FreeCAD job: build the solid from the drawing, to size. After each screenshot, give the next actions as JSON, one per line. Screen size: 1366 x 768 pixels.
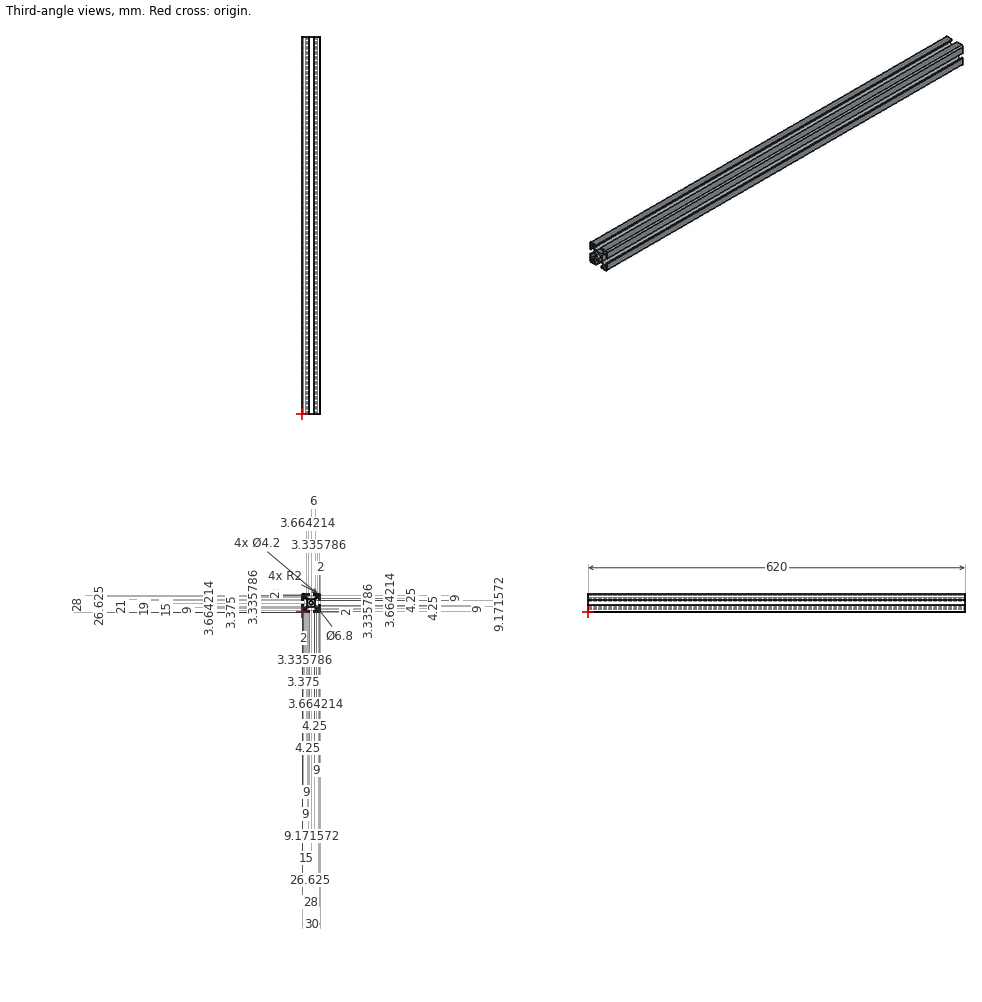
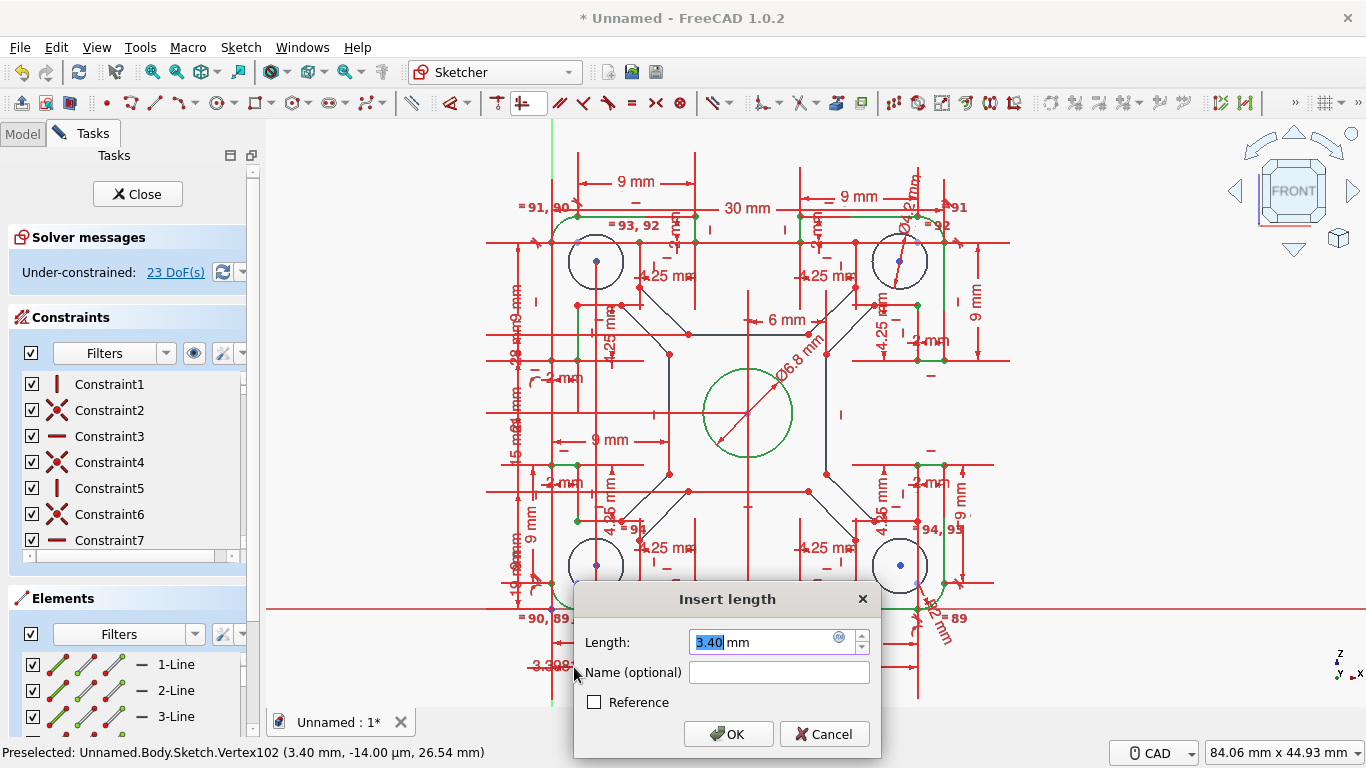
{"action": "type", "text": "3.375"}
{"action": "key", "text": "Return"}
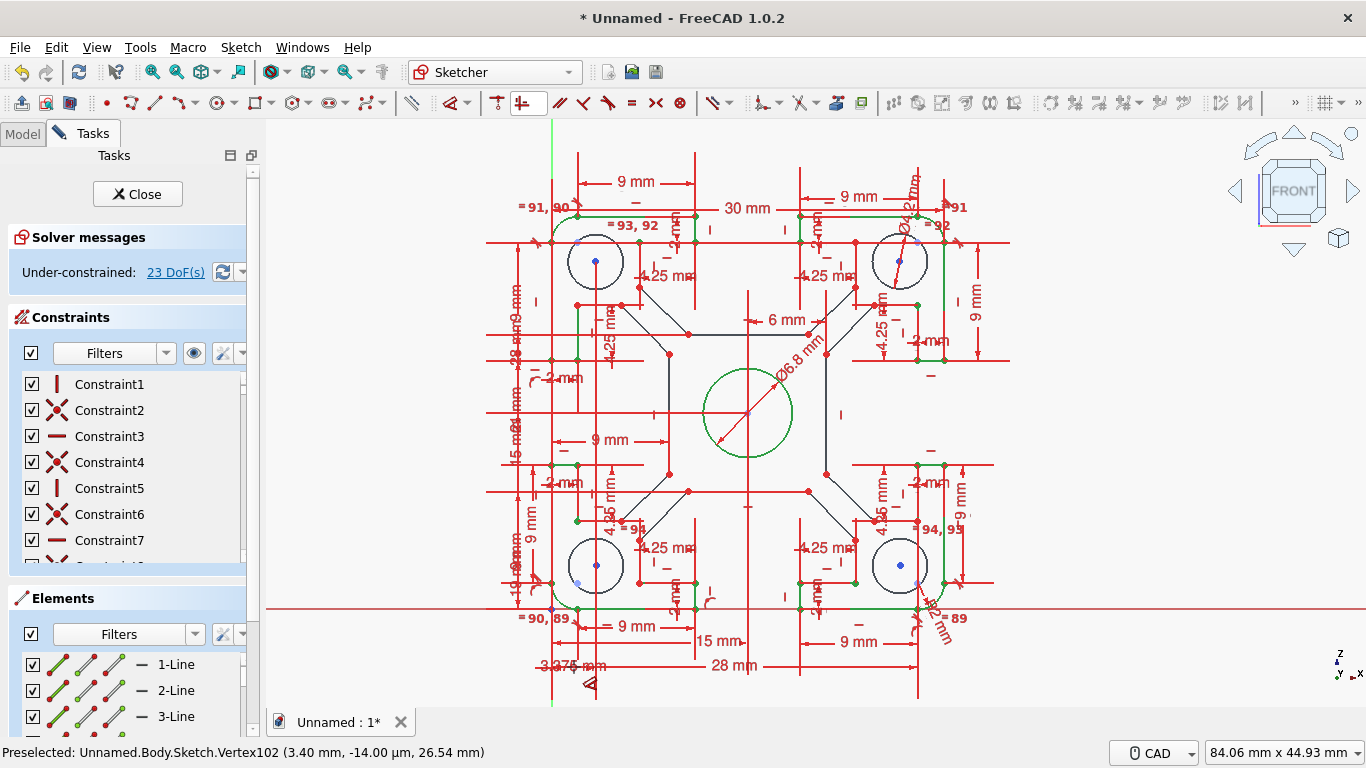
{"action": "left_click", "coordinate": [900, 566]}
{"action": "left_click", "coordinate": [958, 588]}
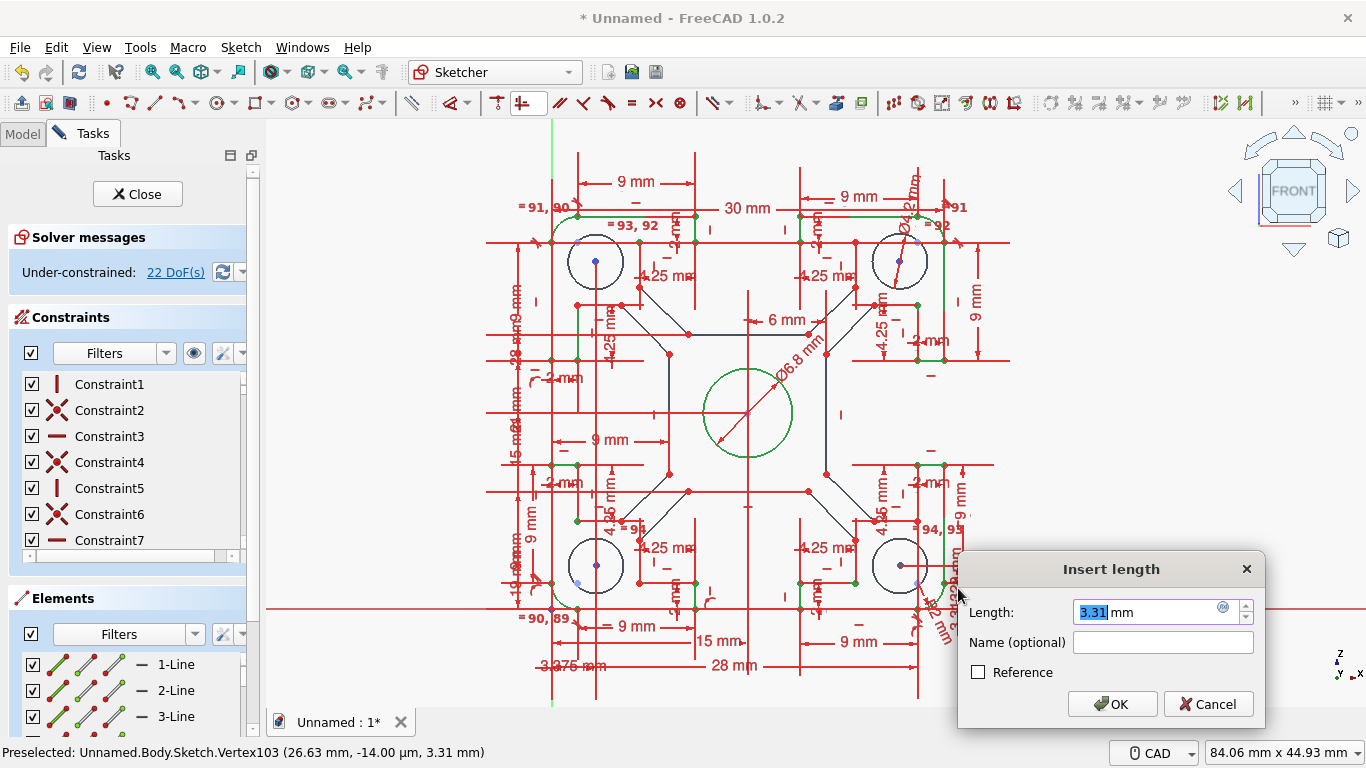
{"action": "type", "text": "3.375"}
{"action": "key", "text": "Return"}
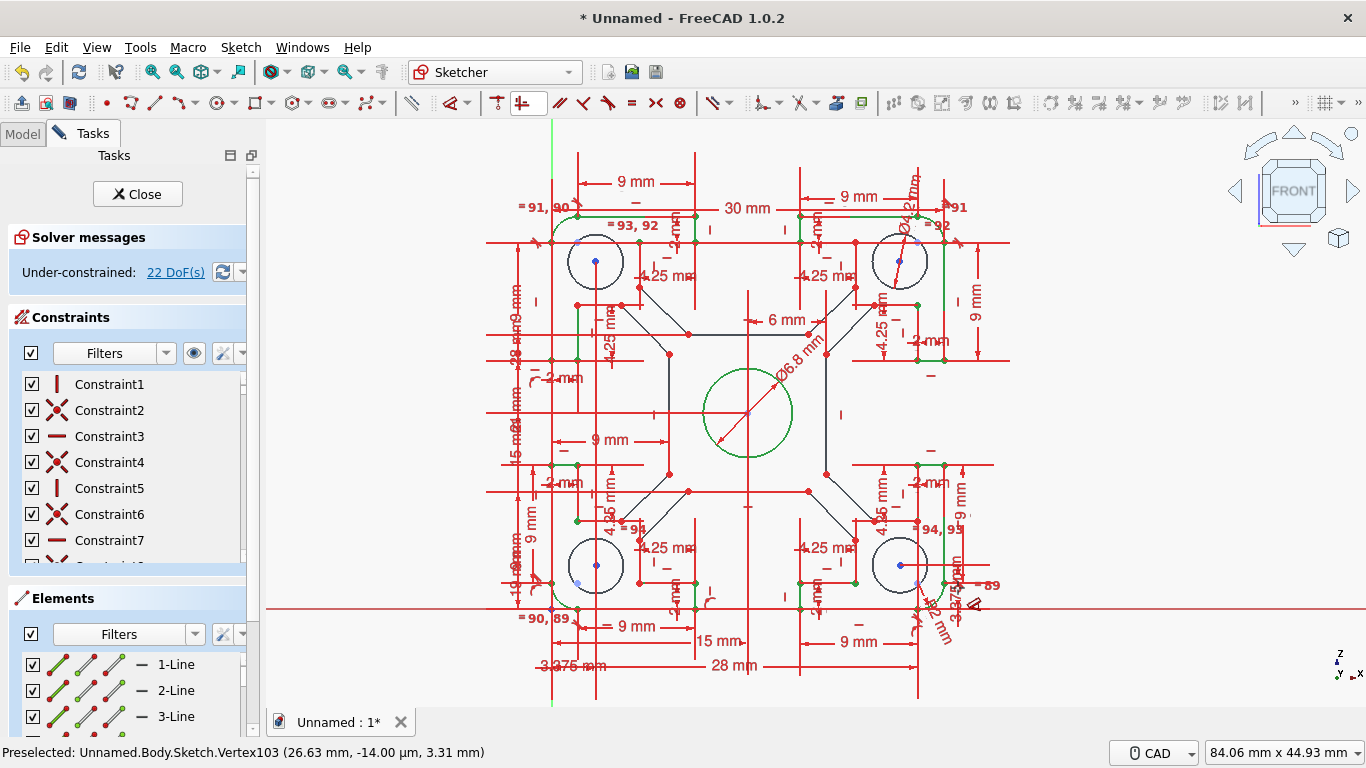
{"action": "left_click", "coordinate": [596, 566]}
{"action": "left_click", "coordinate": [589, 412]}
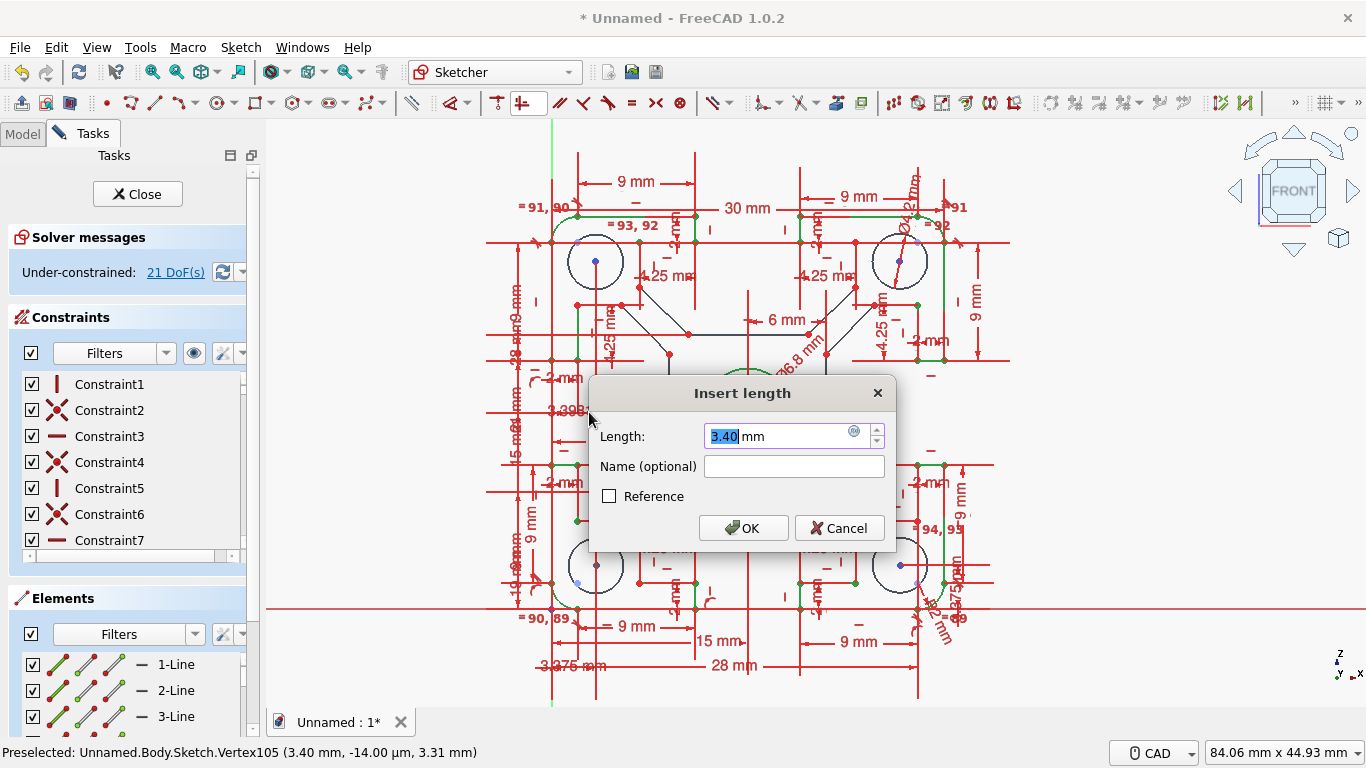
{"action": "type", "text": "3.375"}
{"action": "key", "text": "Return"}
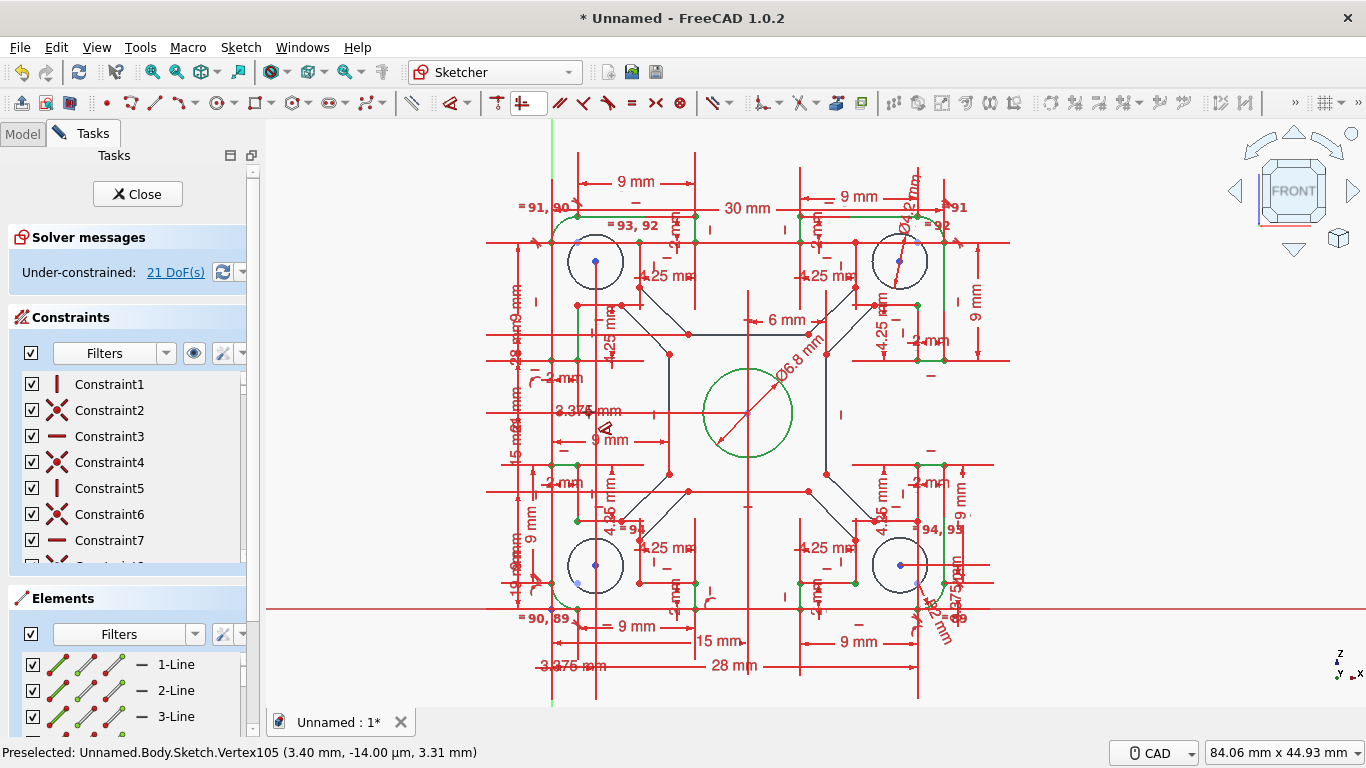
{"action": "left_click", "coordinate": [596, 566]}
{"action": "left_click", "coordinate": [446, 588]}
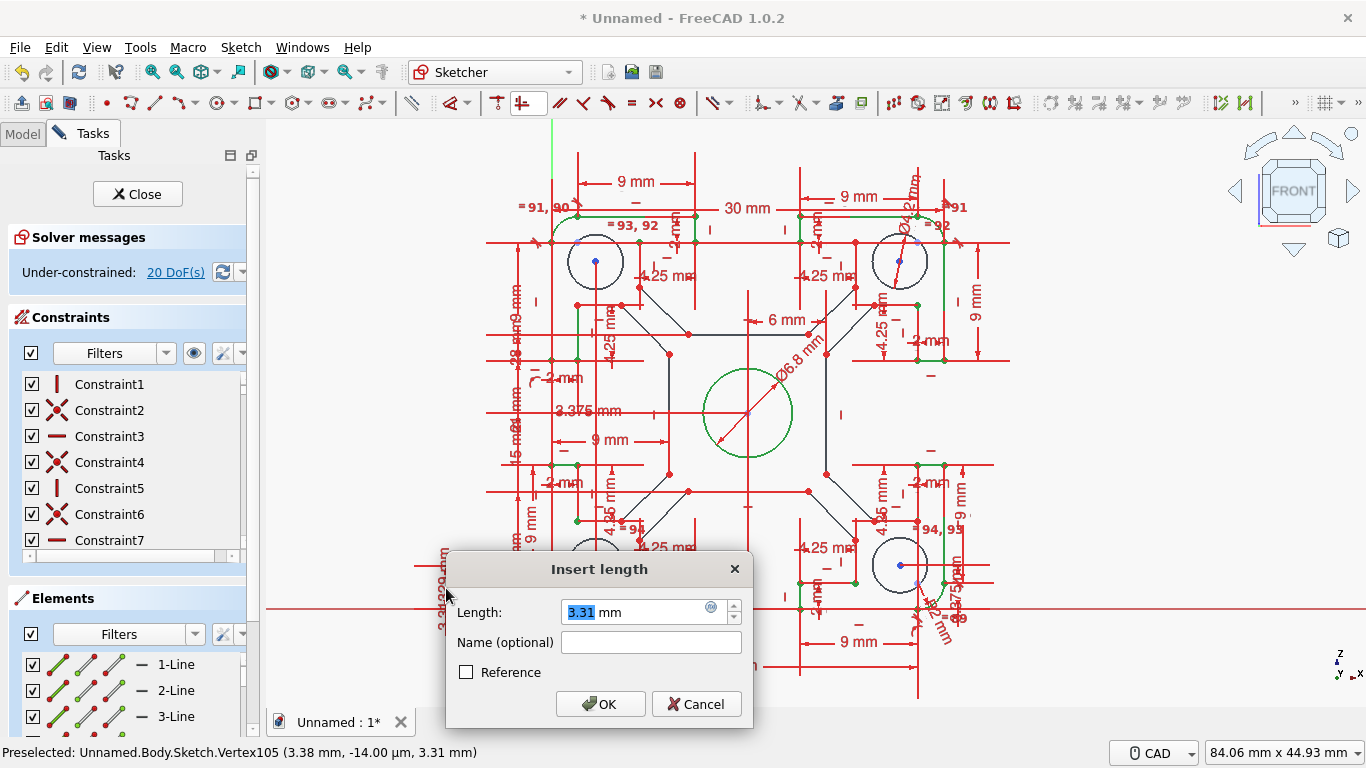
{"action": "type", "text": "3.375"}
{"action": "key", "text": "Return"}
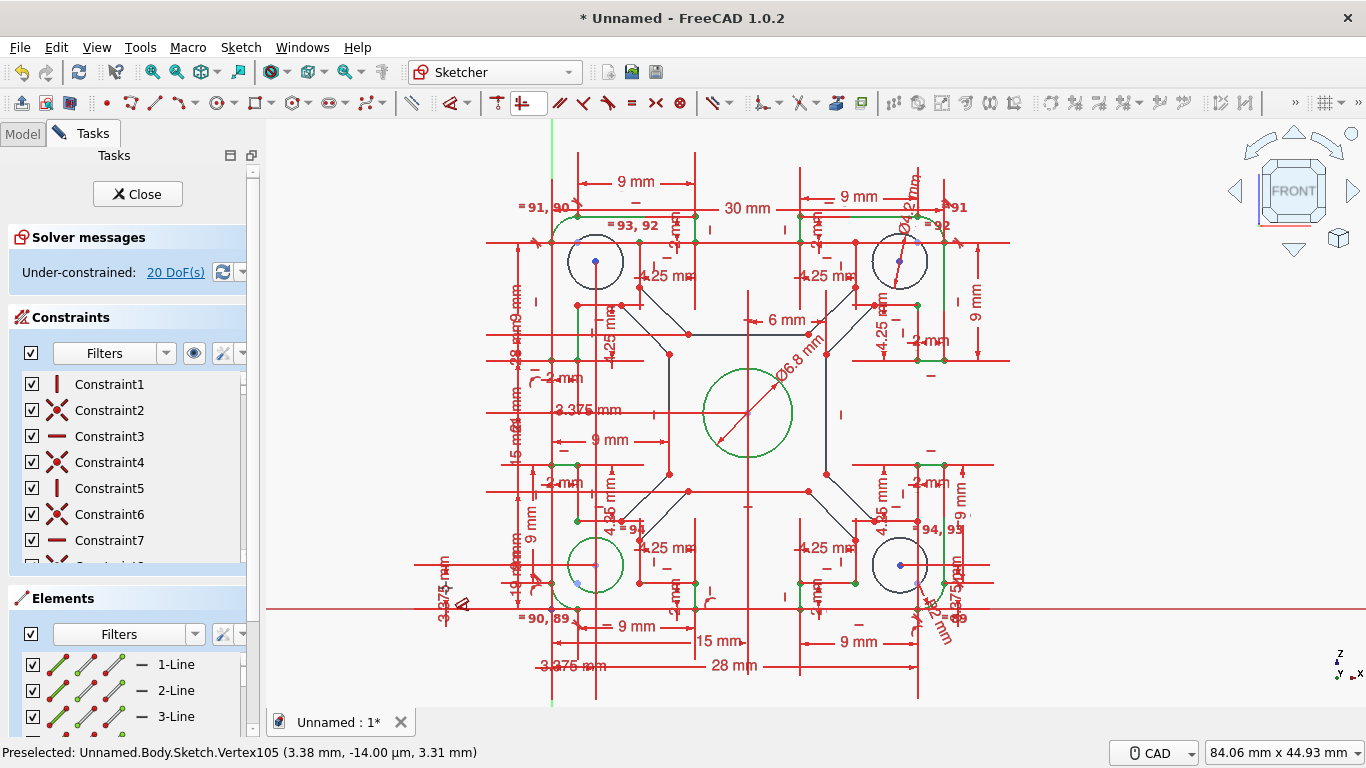
{"action": "left_click", "coordinate": [900, 261]}
{"action": "left_click", "coordinate": [646, 667]}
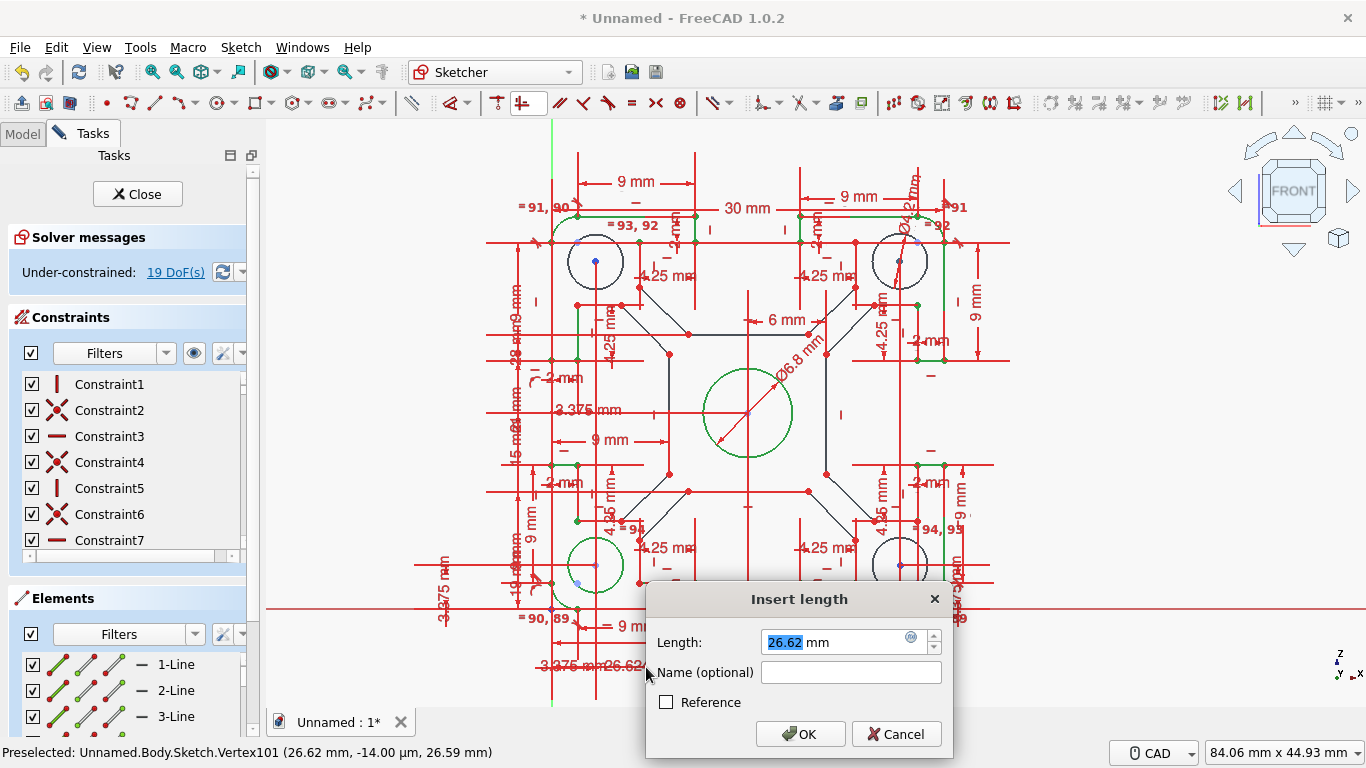
{"action": "type", "text": "26.625"}
{"action": "key", "text": "Return"}